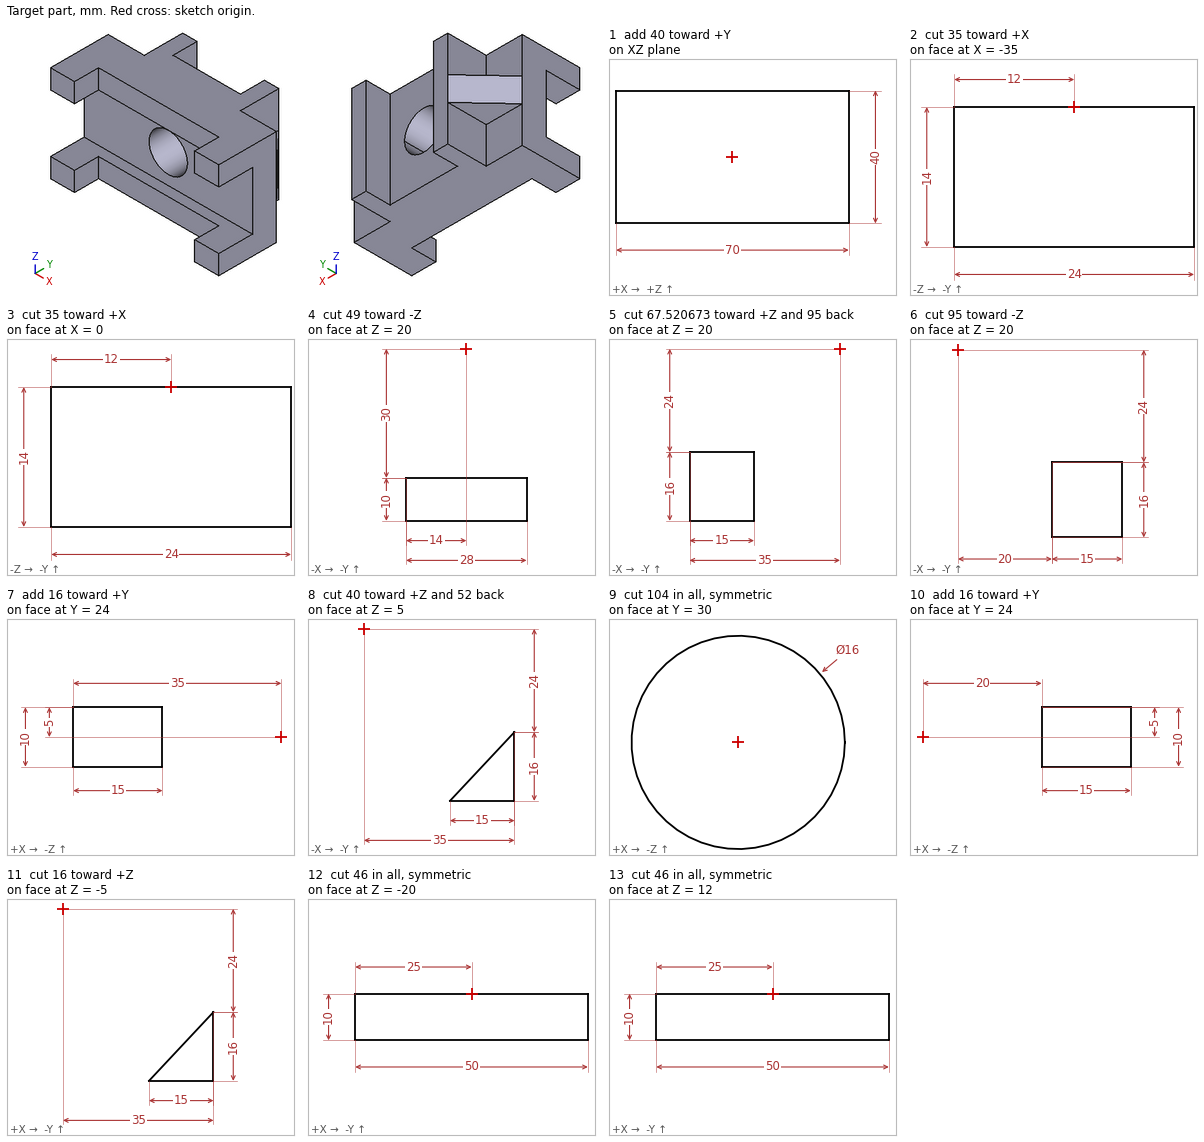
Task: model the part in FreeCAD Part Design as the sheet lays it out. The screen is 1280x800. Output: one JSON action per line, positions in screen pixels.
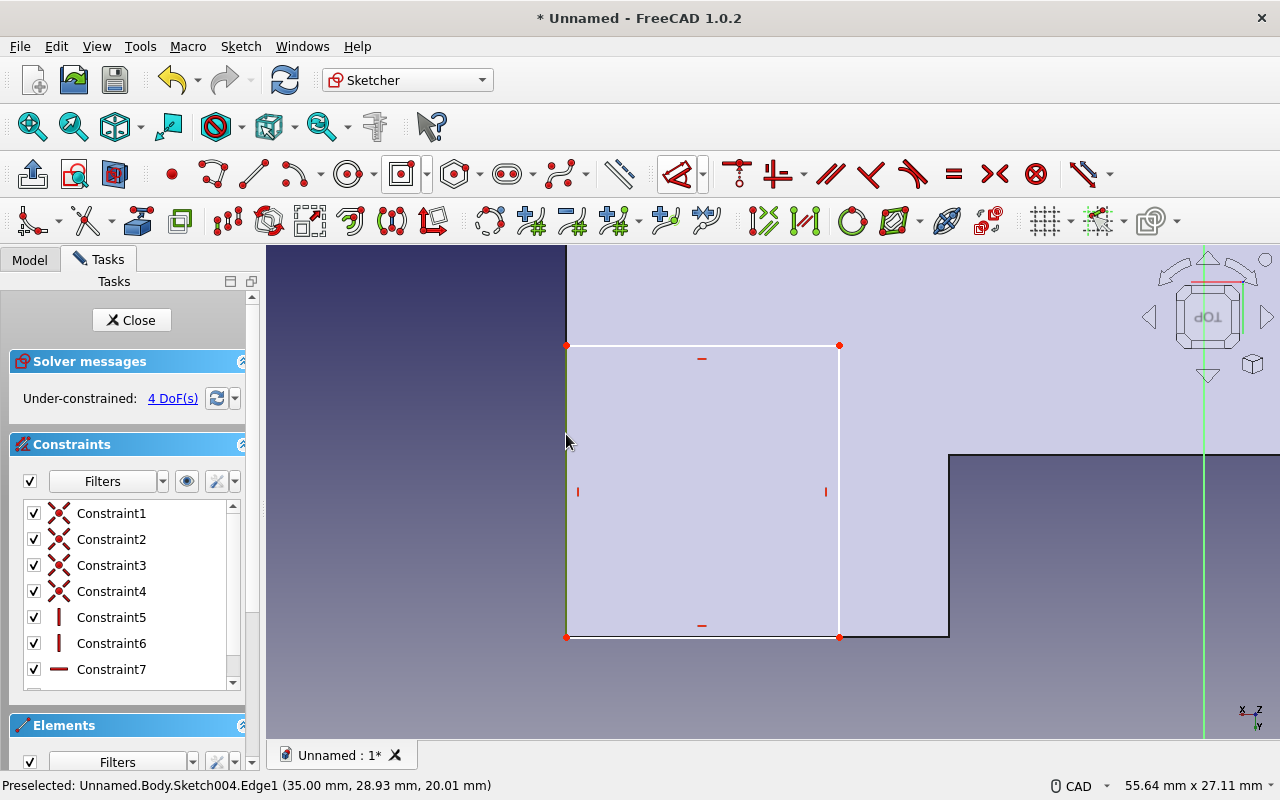
{"action": "key", "text": "i"}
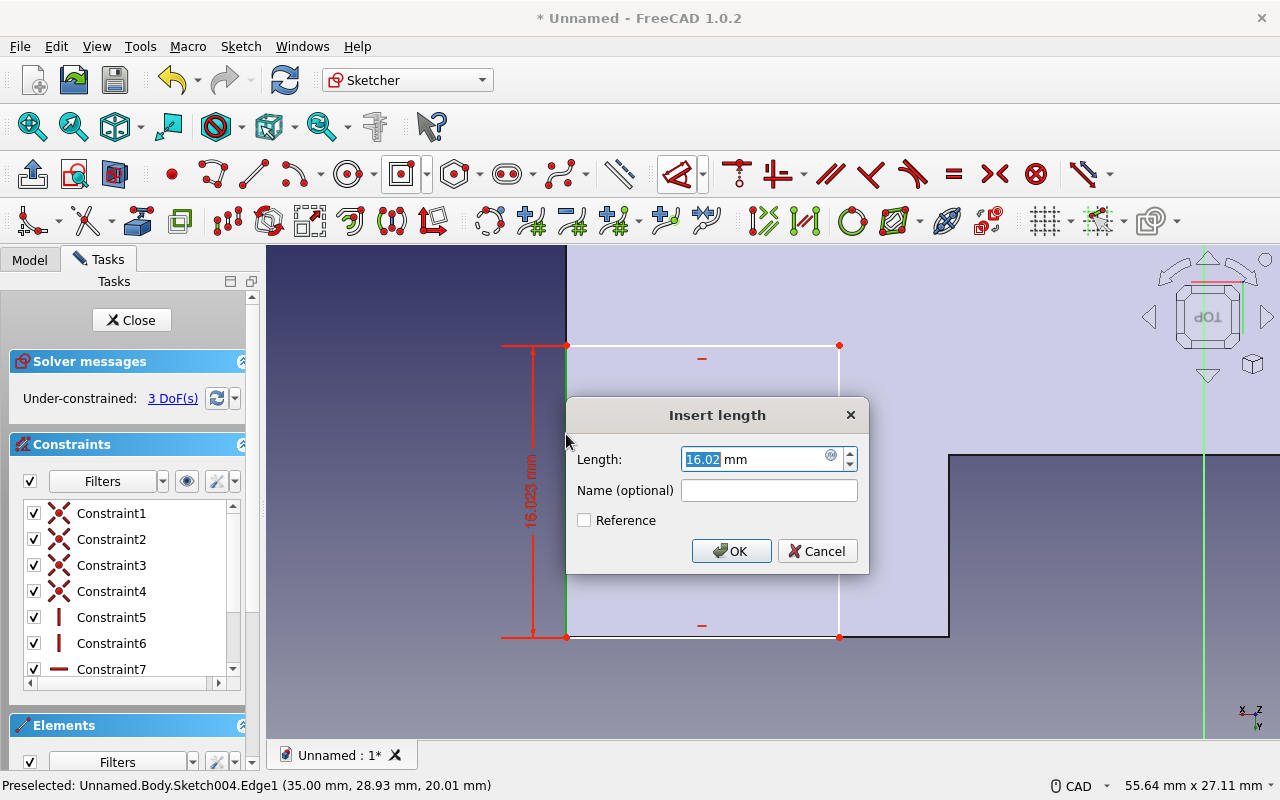
{"action": "type", "text": "16"}
{"action": "key", "text": "Return"}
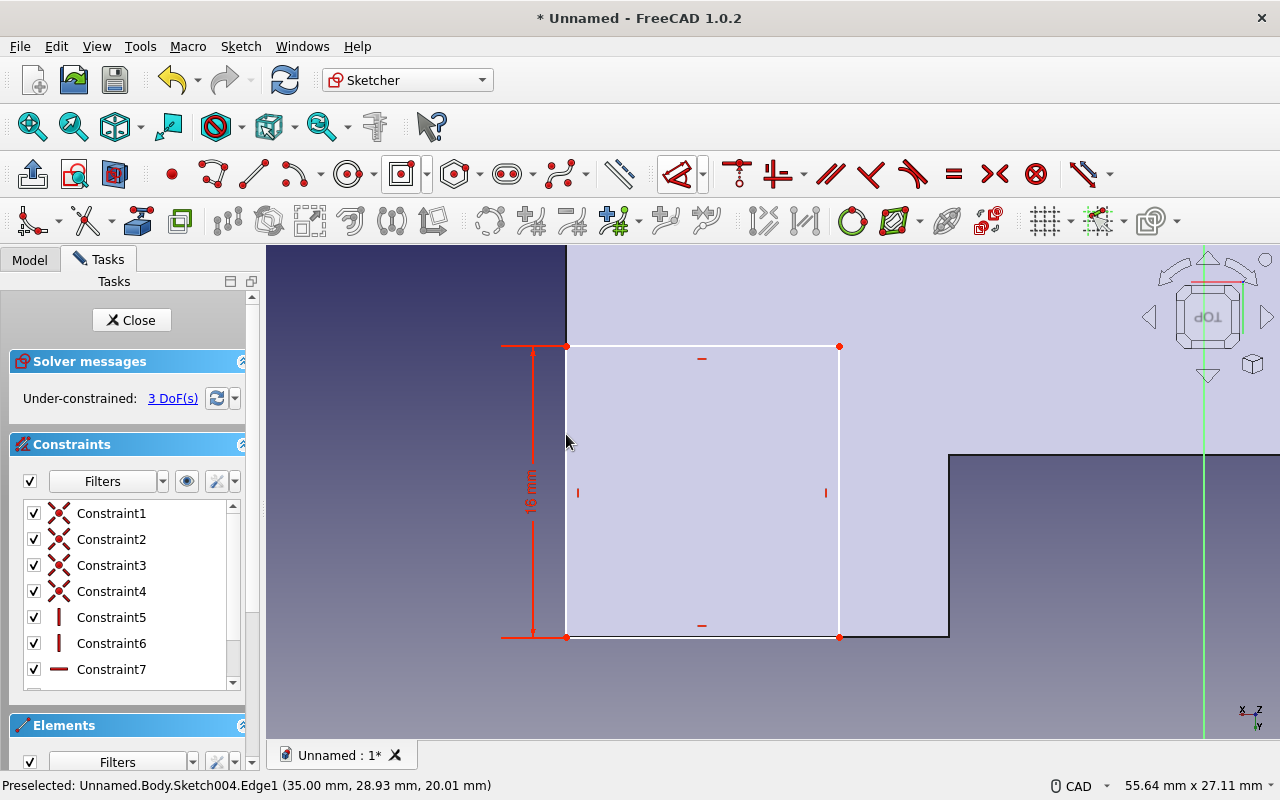
{"action": "left_click", "coordinate": [648, 638]}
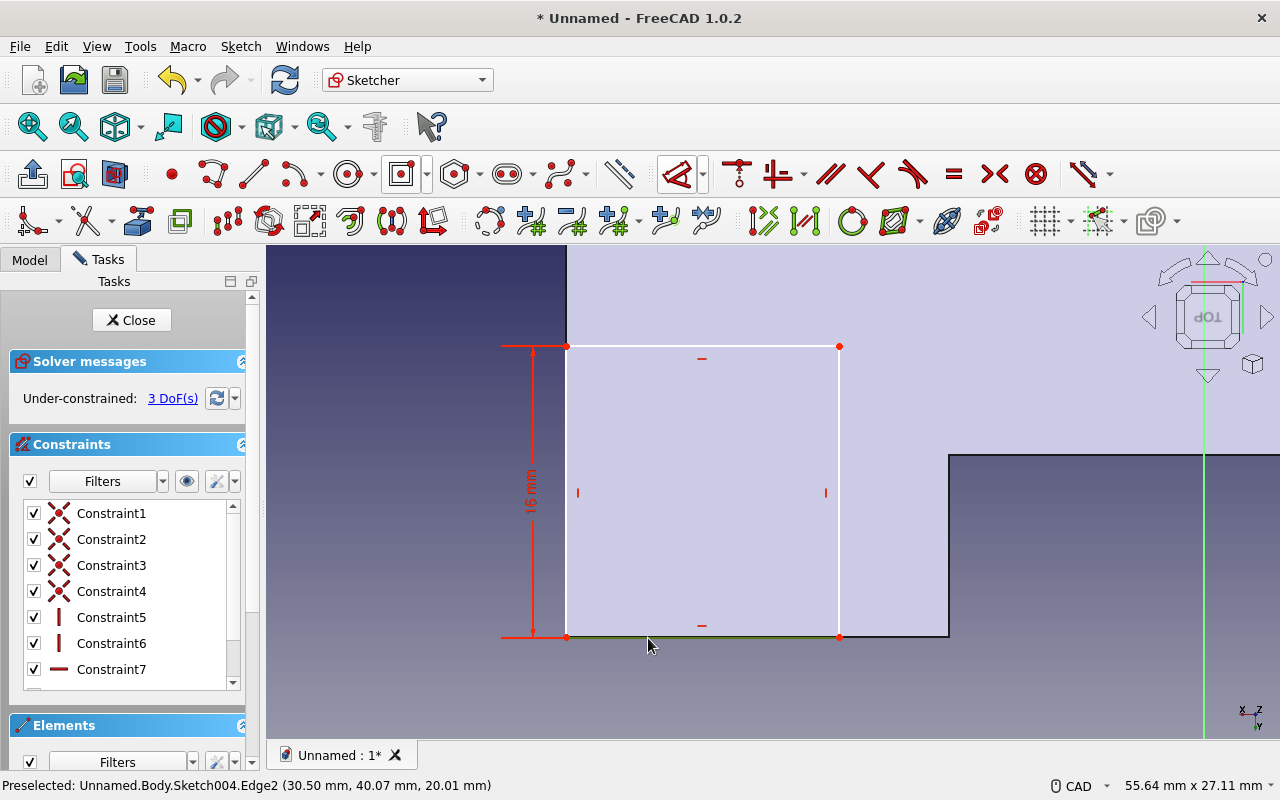
{"action": "key", "text": "l"}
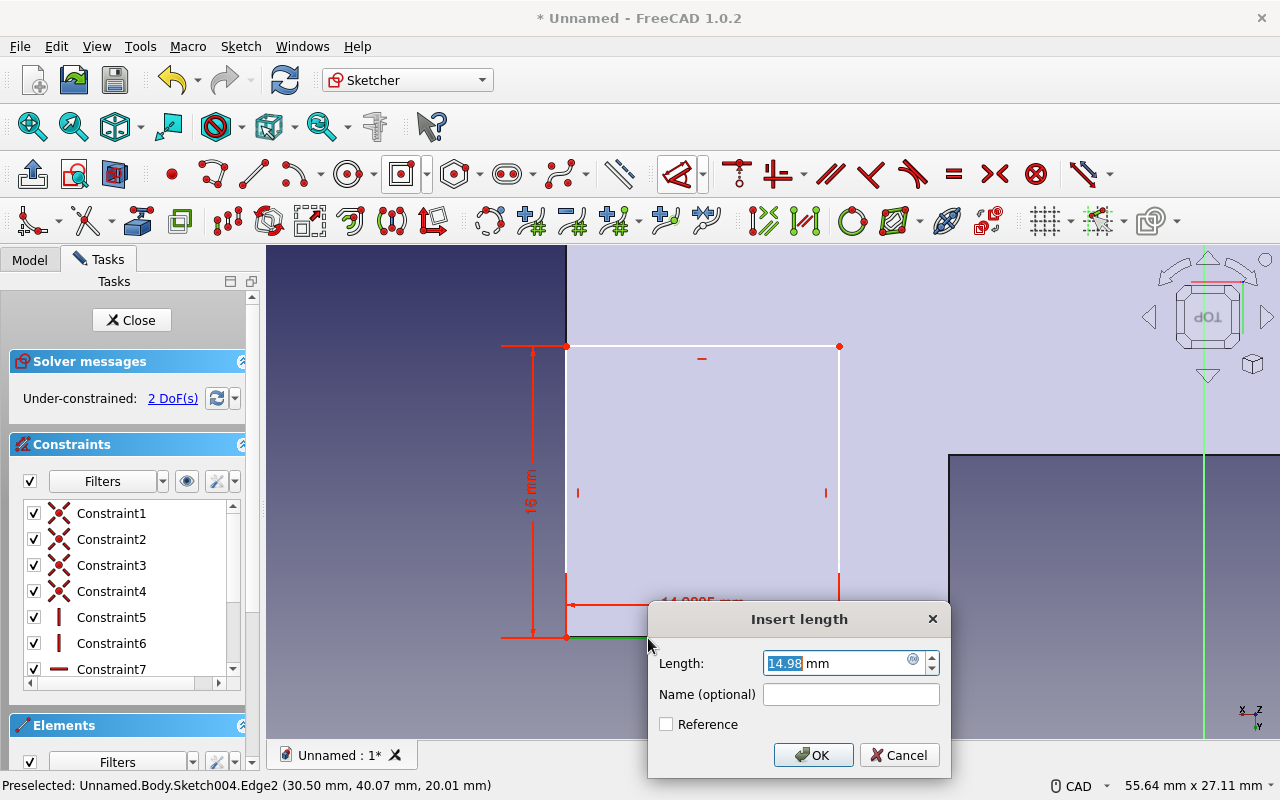
{"action": "type", "text": "15"}
{"action": "key", "text": "Return"}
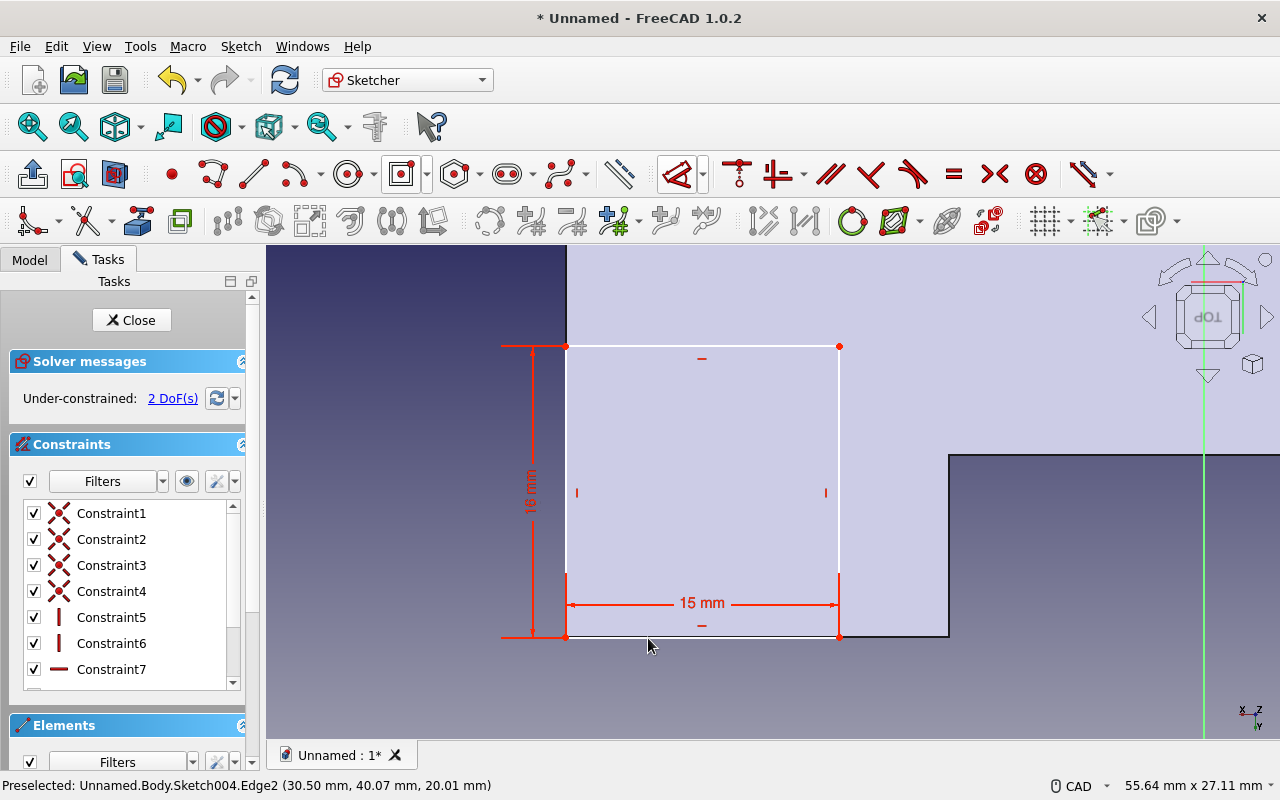
{"action": "left_click", "coordinate": [566, 346]}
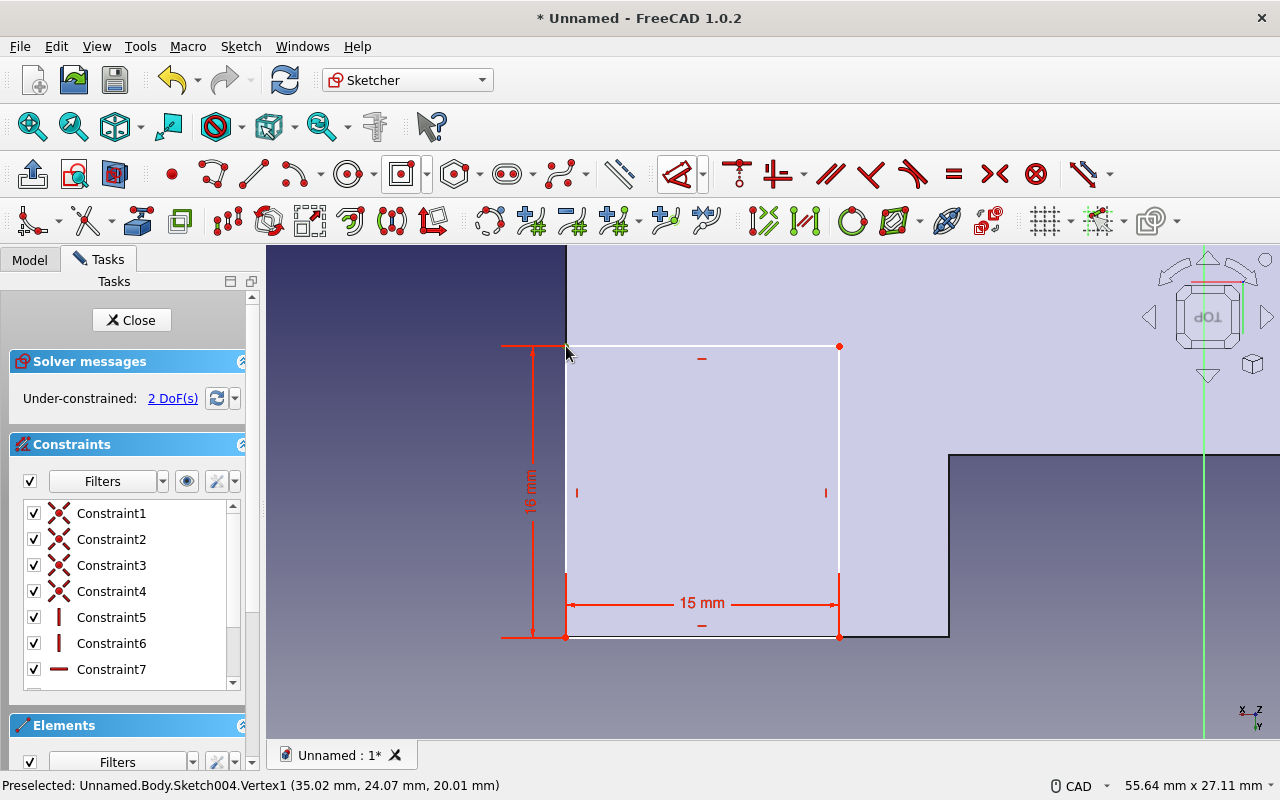
{"action": "key", "text": "l"}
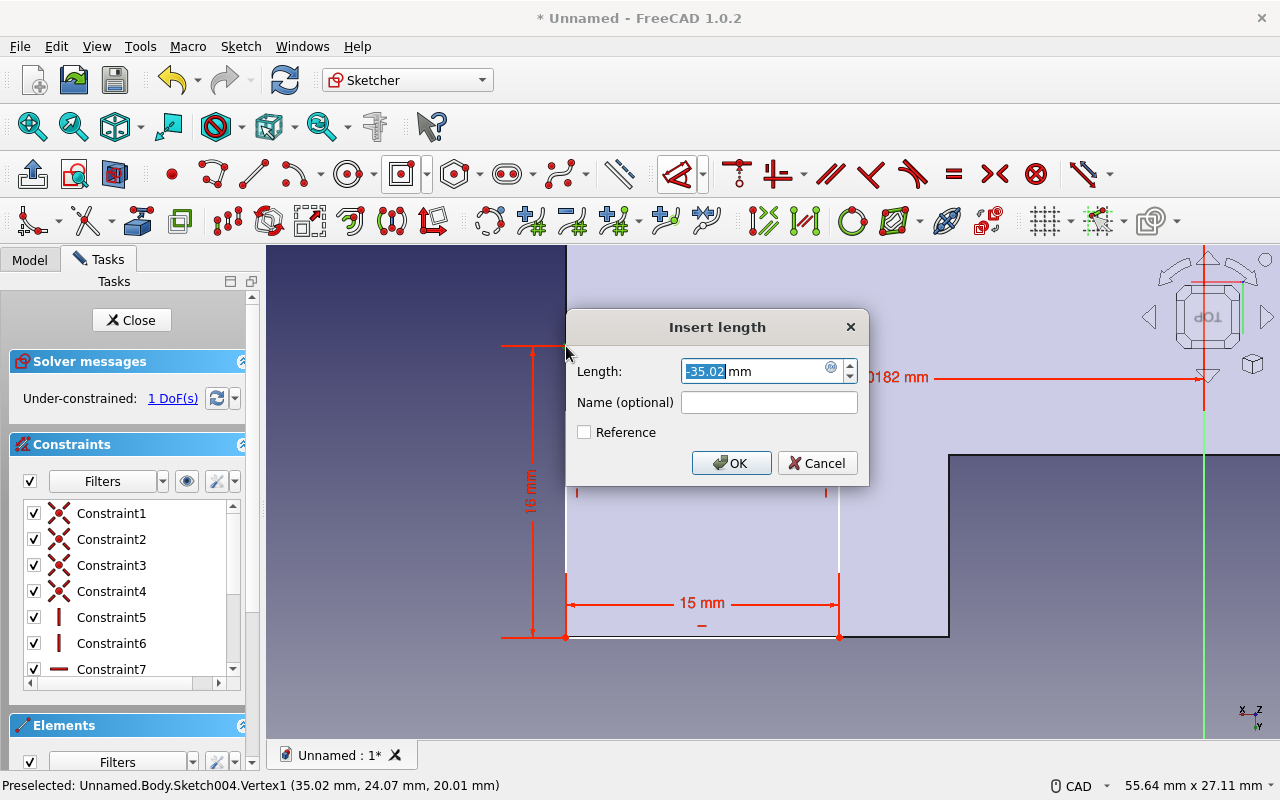
{"action": "type", "text": "-35"}
{"action": "key", "text": "Return"}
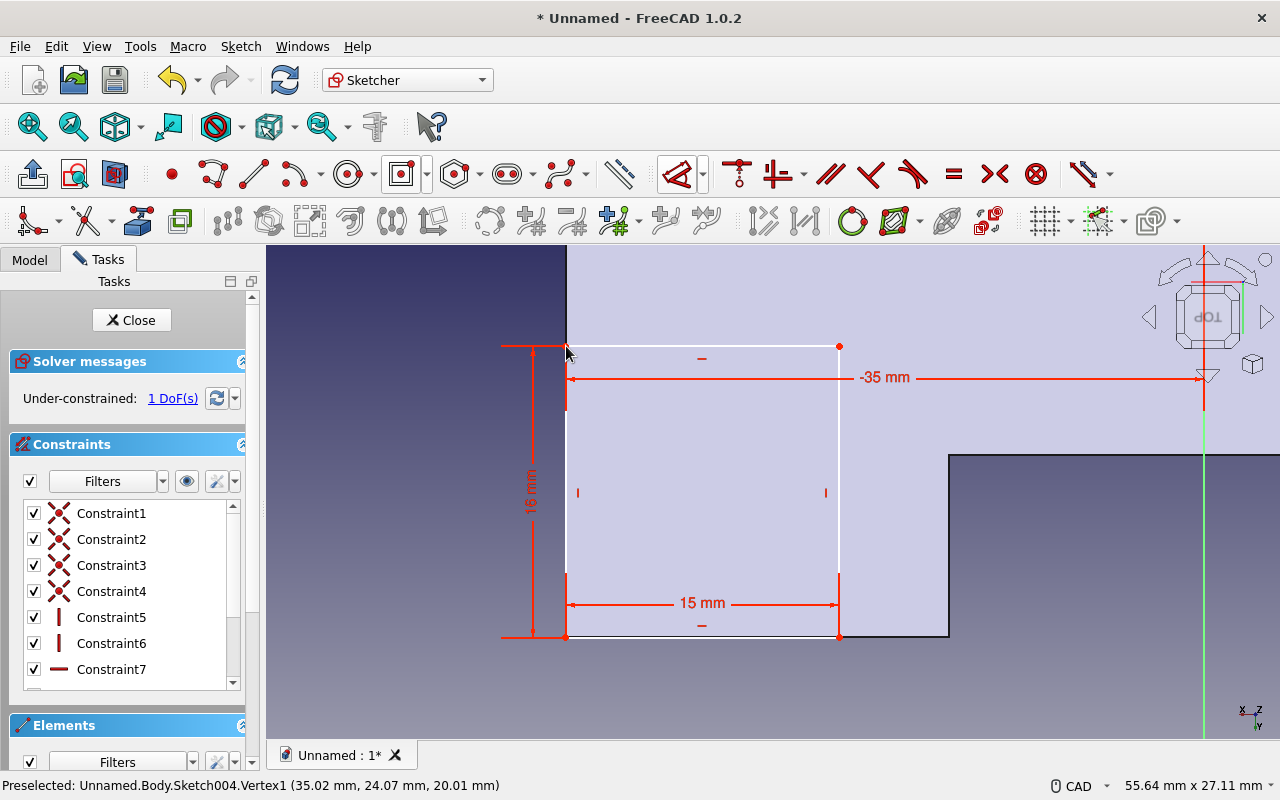
{"action": "left_click", "coordinate": [566, 346]}